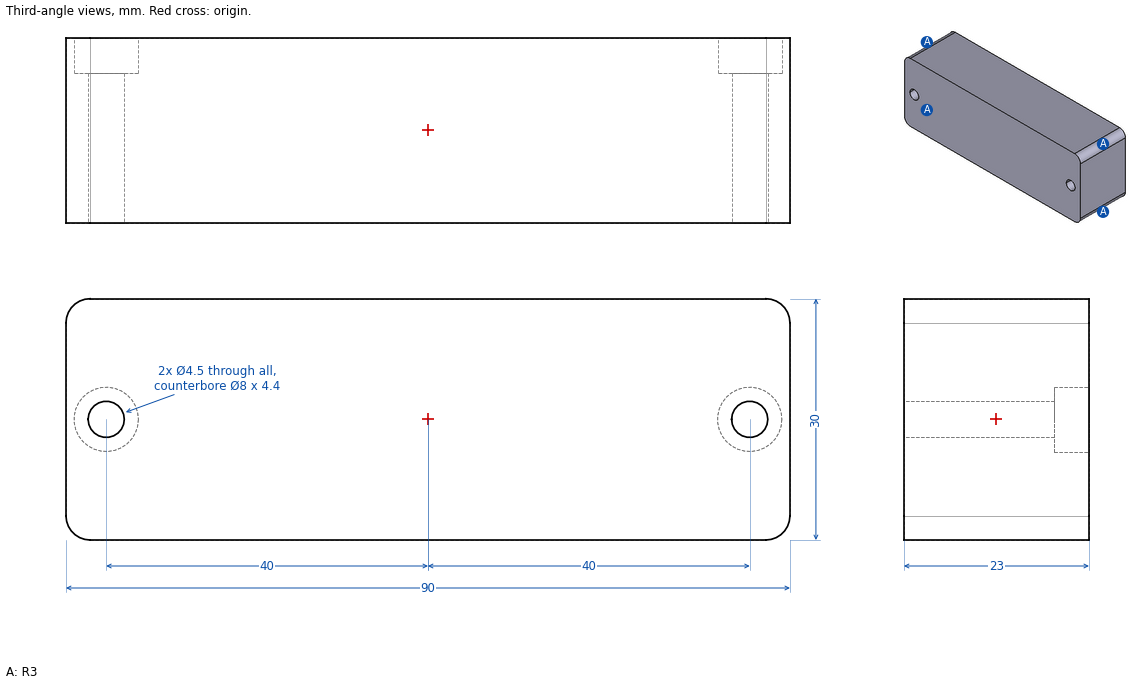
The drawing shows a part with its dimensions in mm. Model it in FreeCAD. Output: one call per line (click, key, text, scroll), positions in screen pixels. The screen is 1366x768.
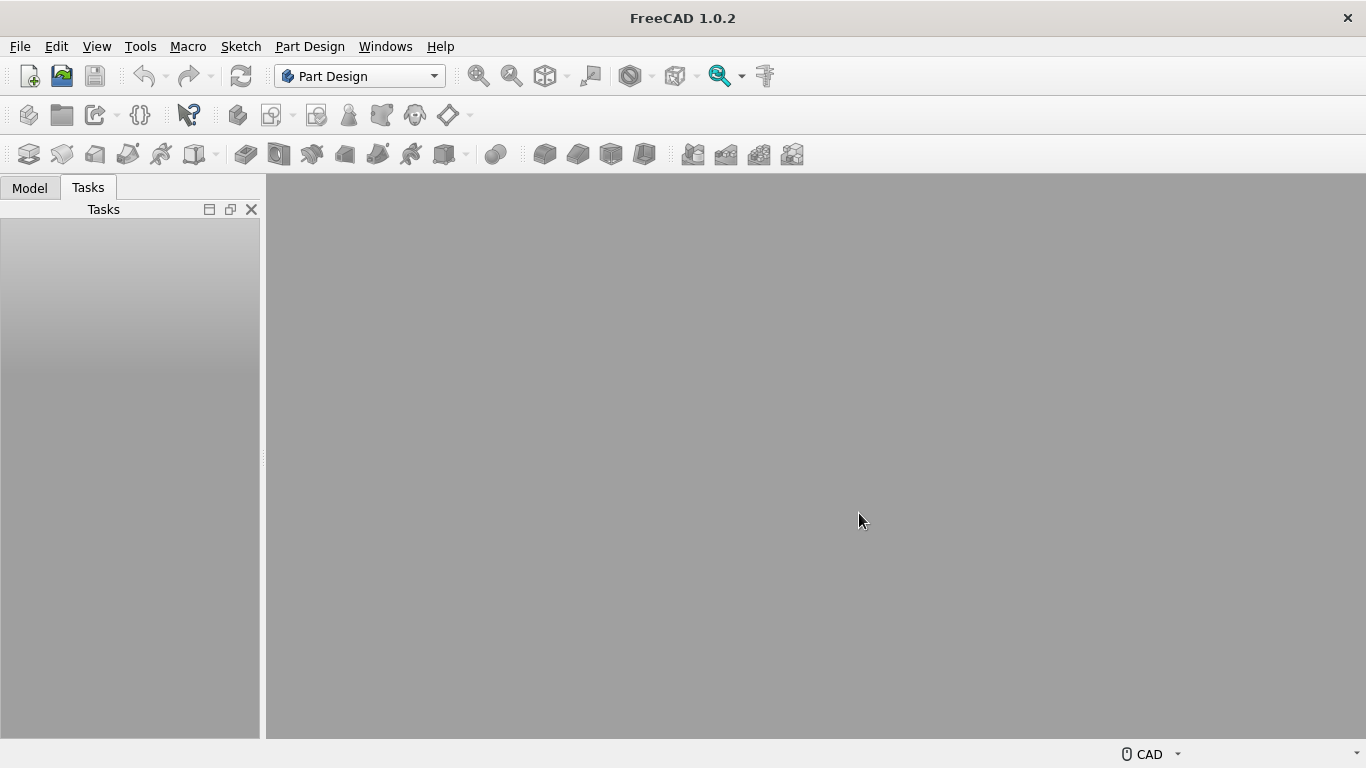
key(ctrl+n)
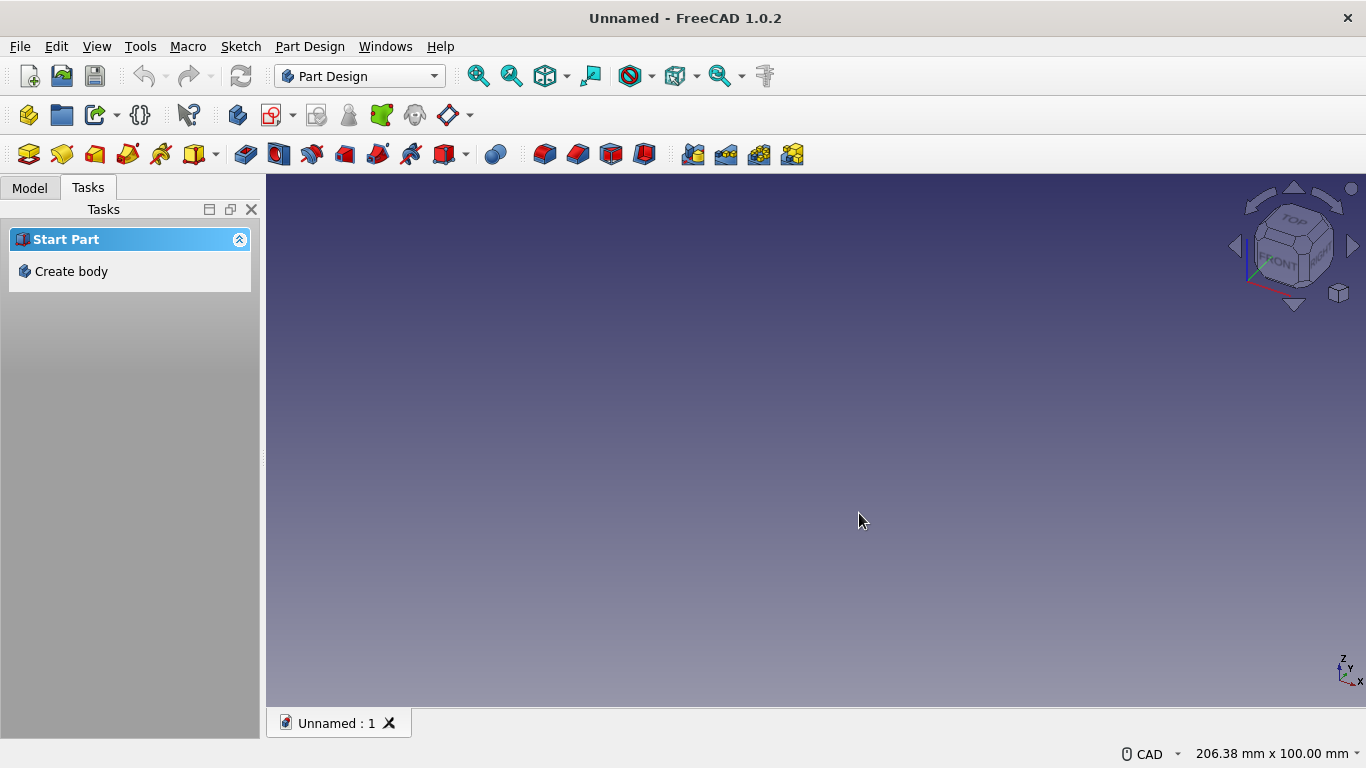
click(270, 116)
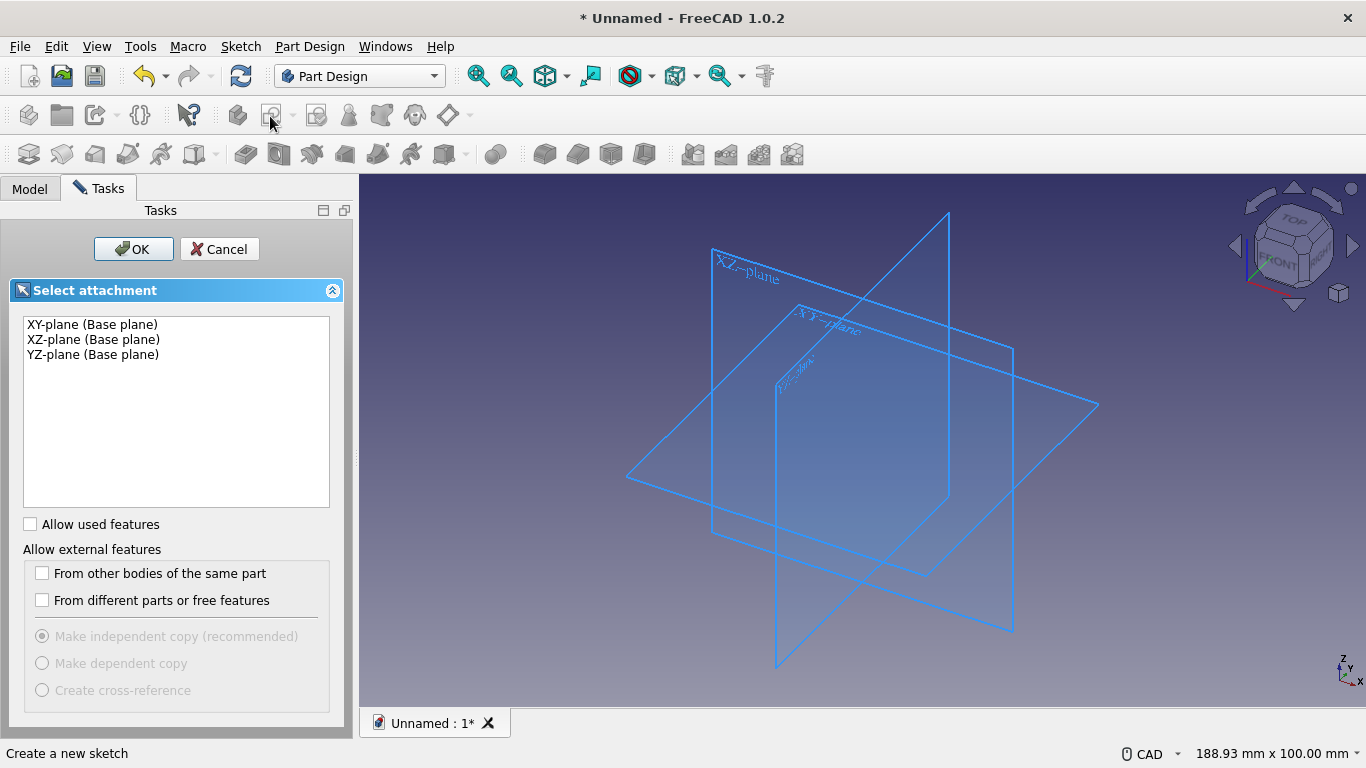
click(84, 340)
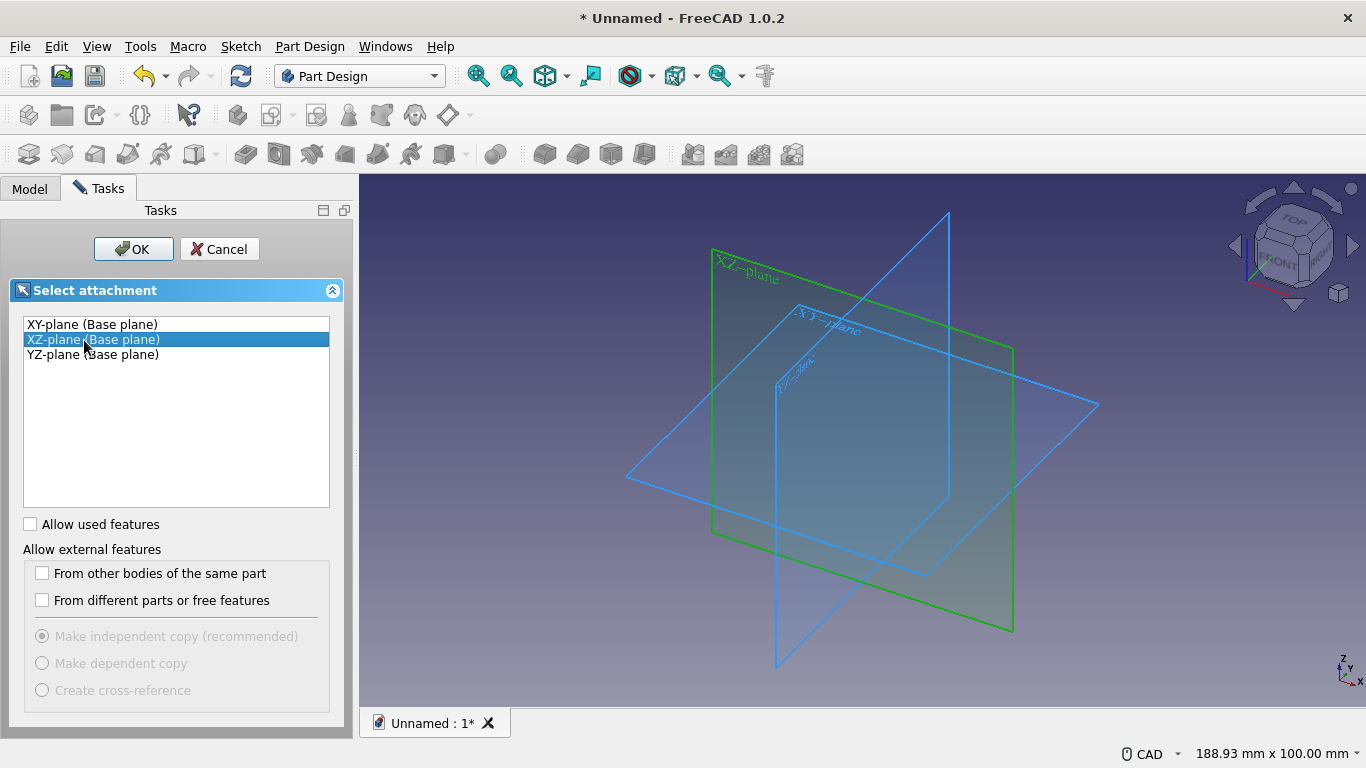
click(134, 249)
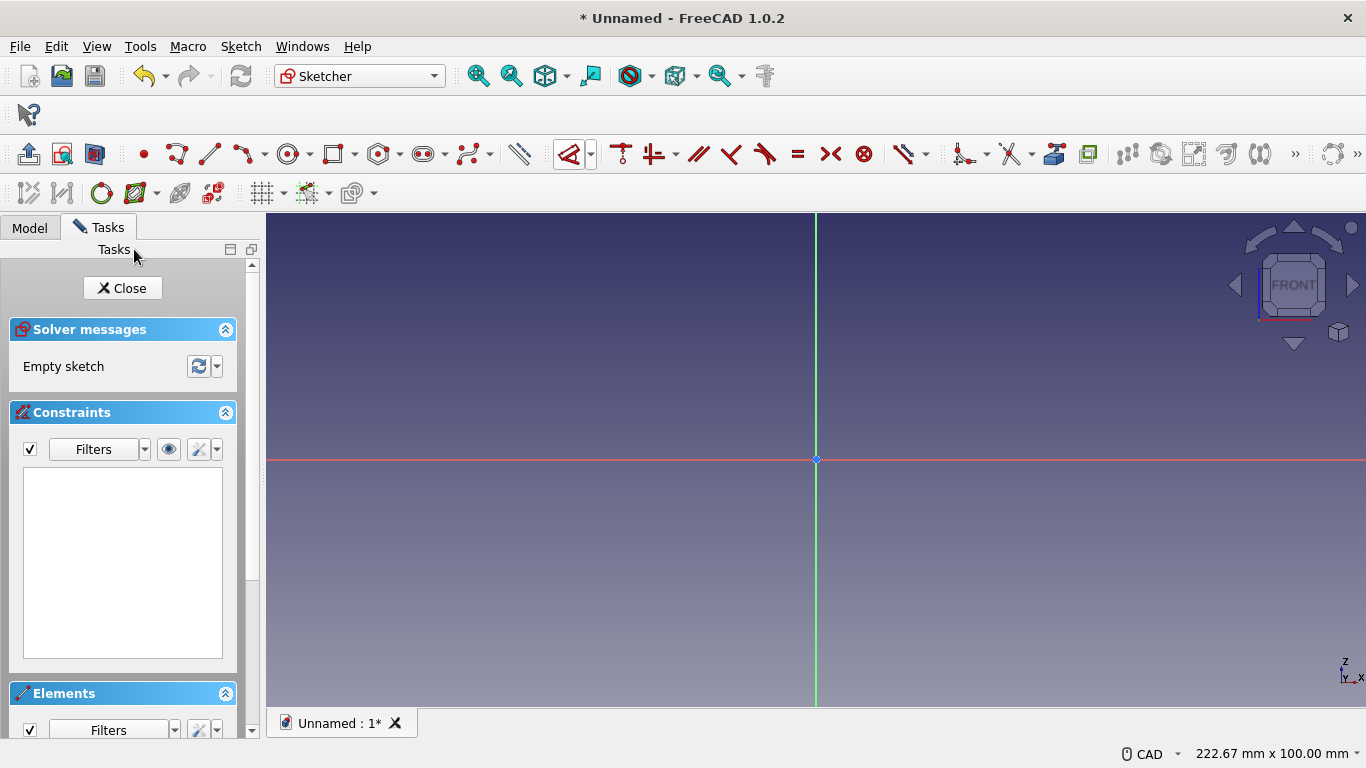
scroll(955, 460, up, 2)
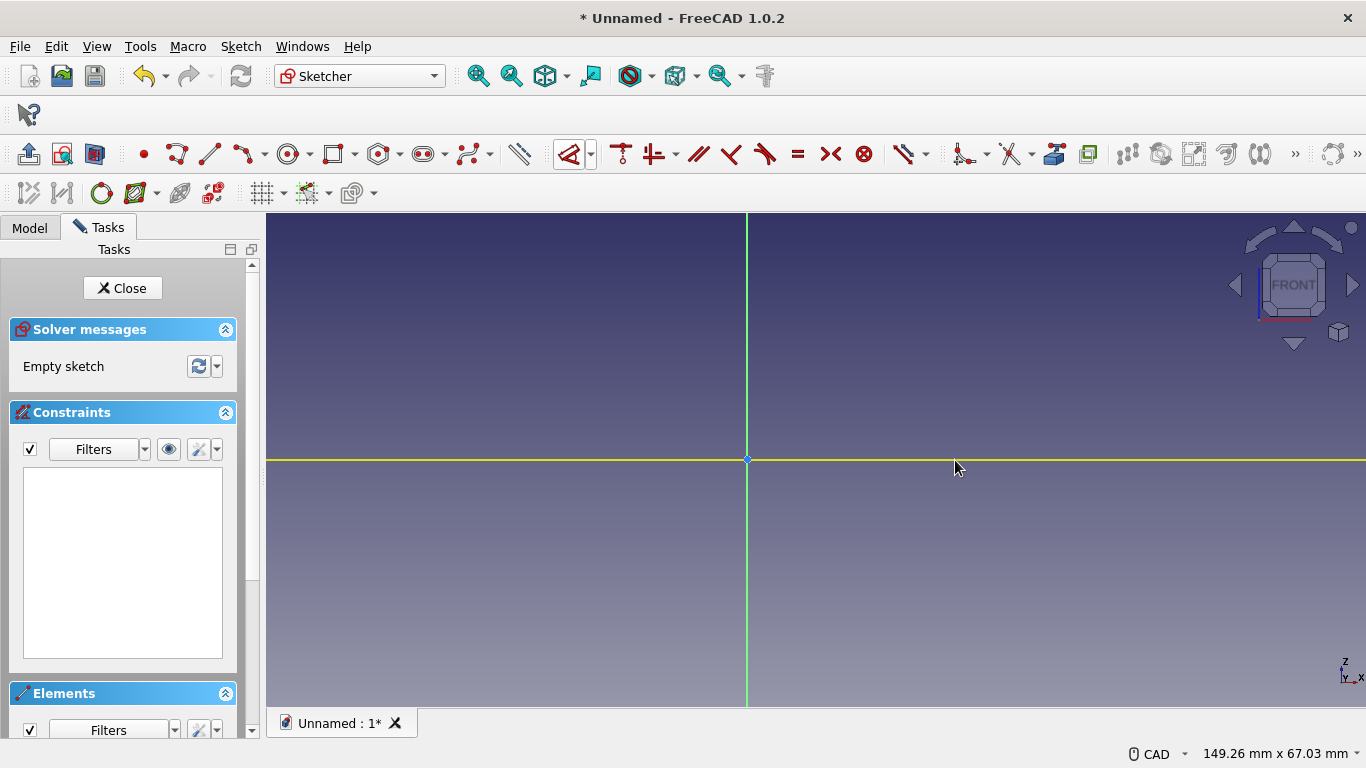
key(g)
key(v)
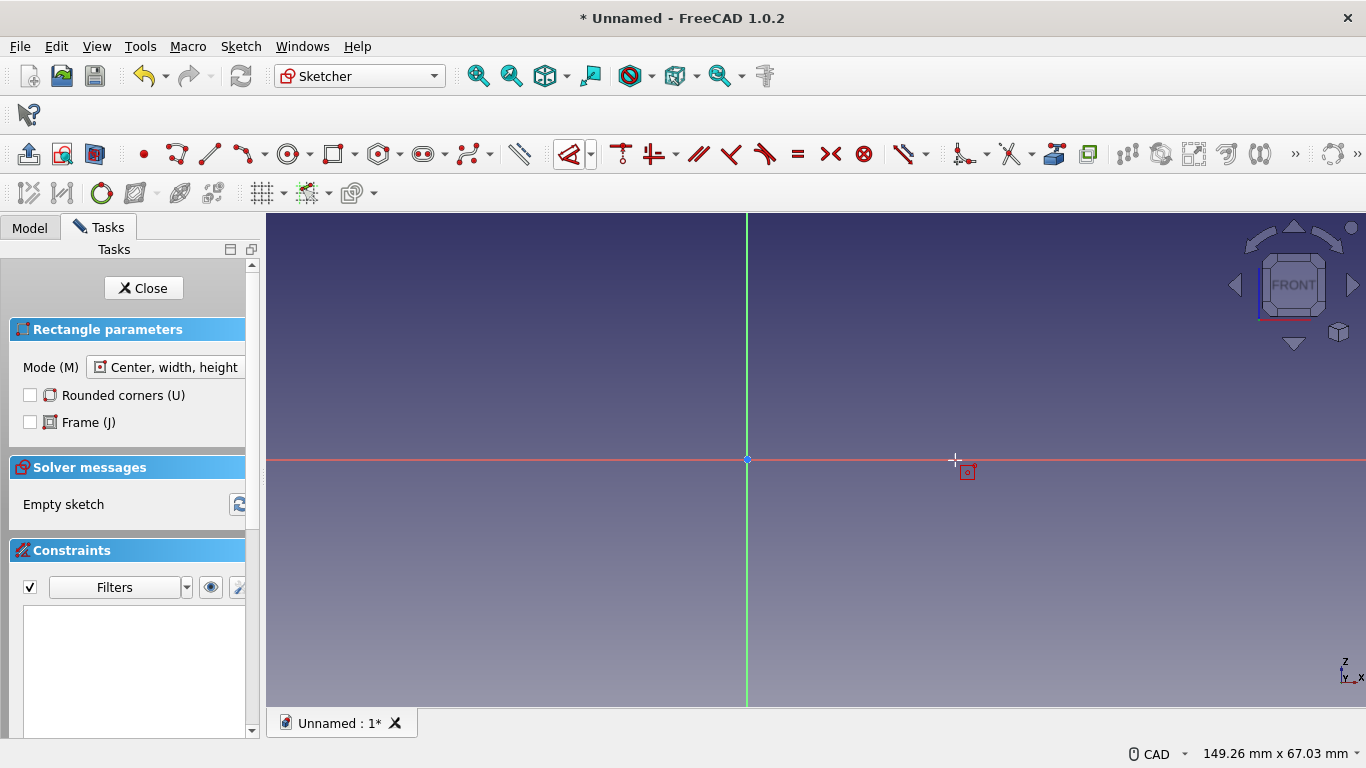
click(747, 460)
move(1079, 349)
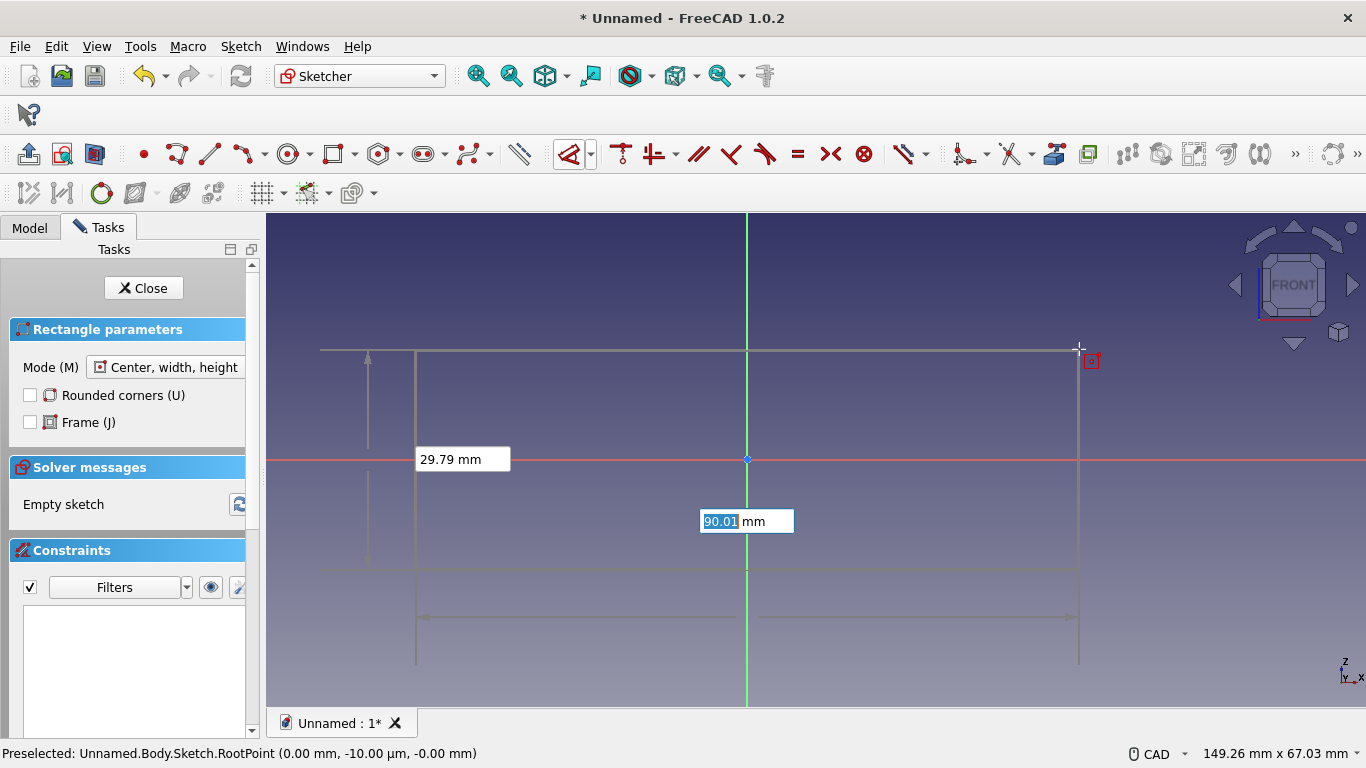
text(90)
key(Tab)
text(30)
key(Return)
key(Escape)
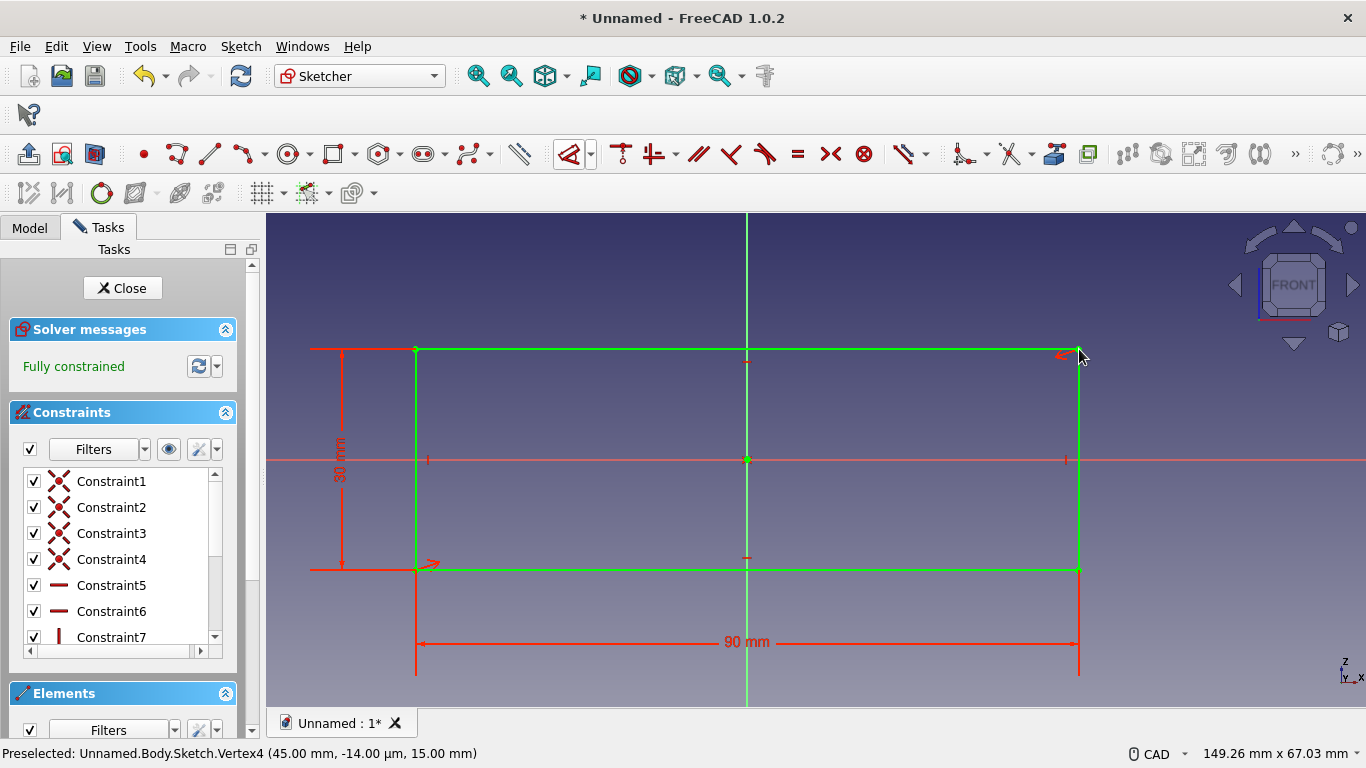
click(123, 288)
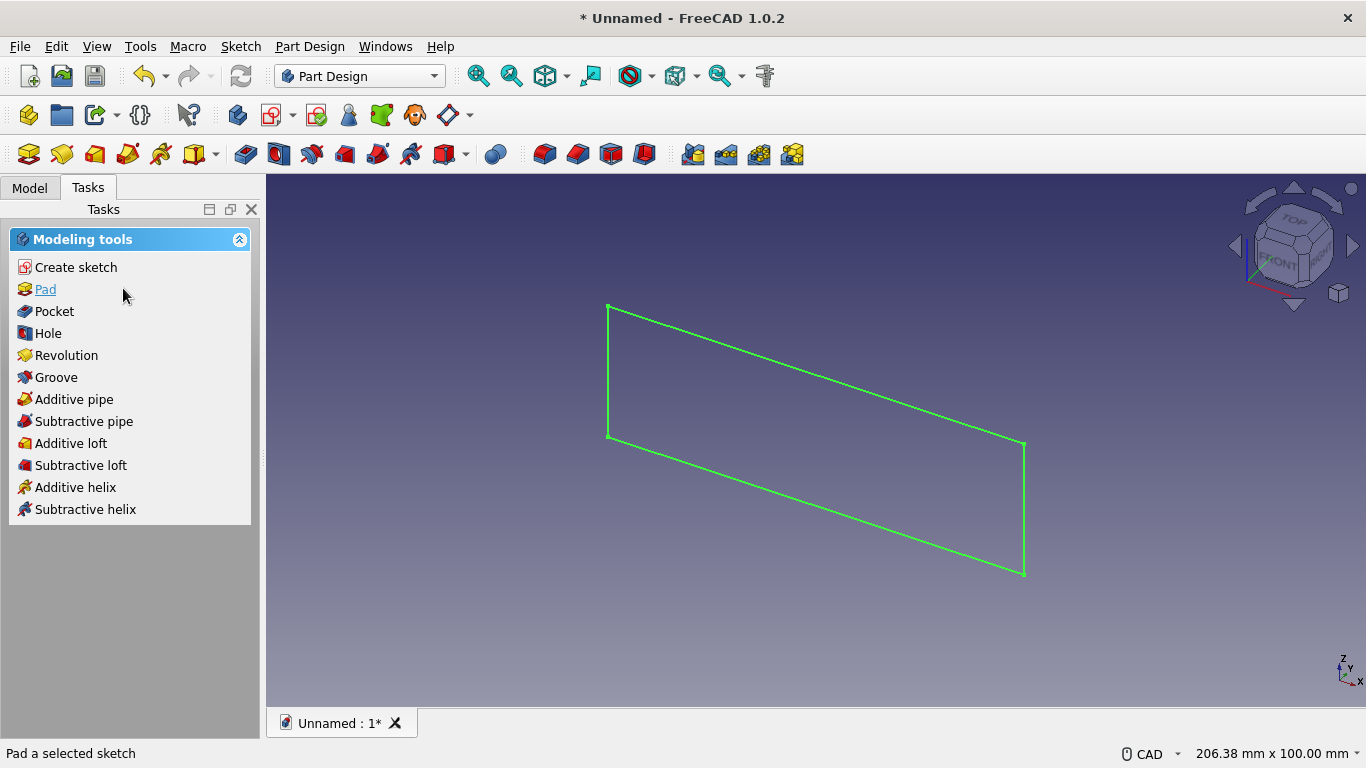
click(29, 154)